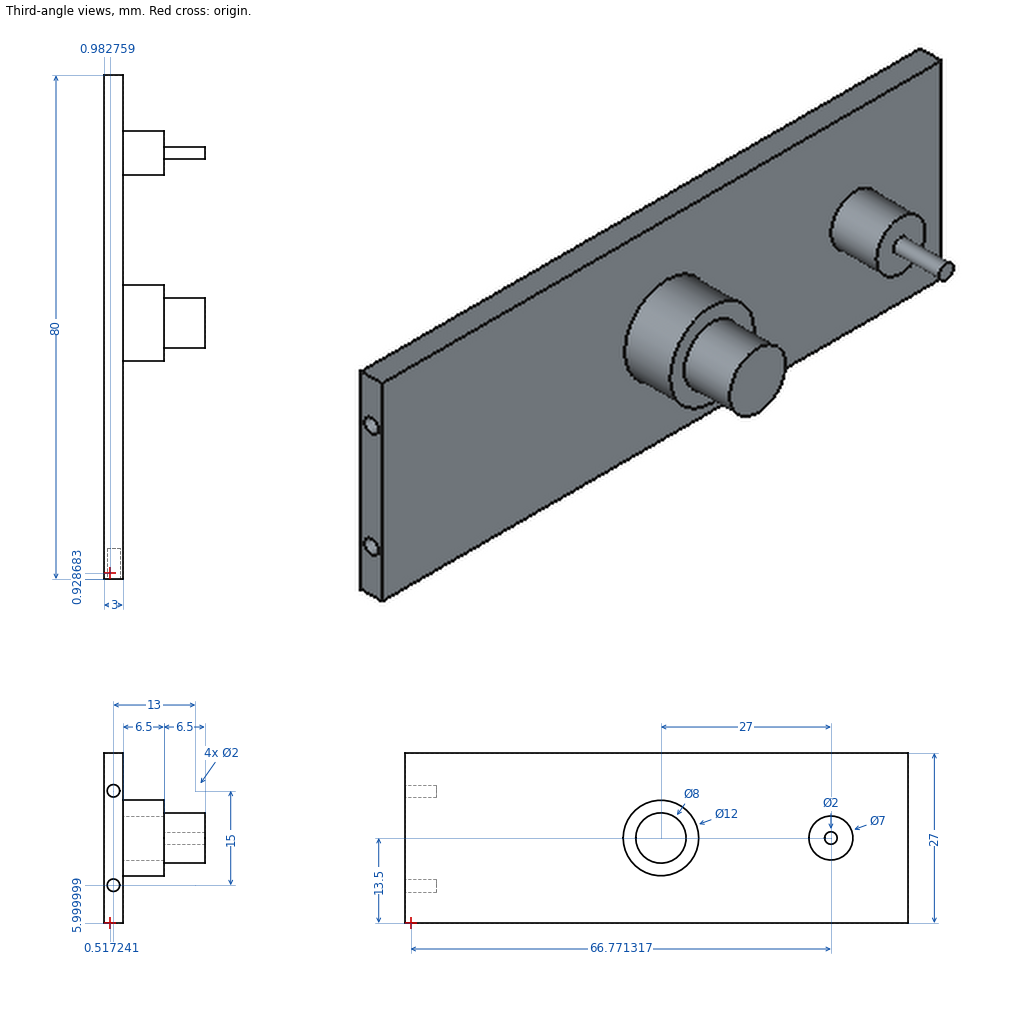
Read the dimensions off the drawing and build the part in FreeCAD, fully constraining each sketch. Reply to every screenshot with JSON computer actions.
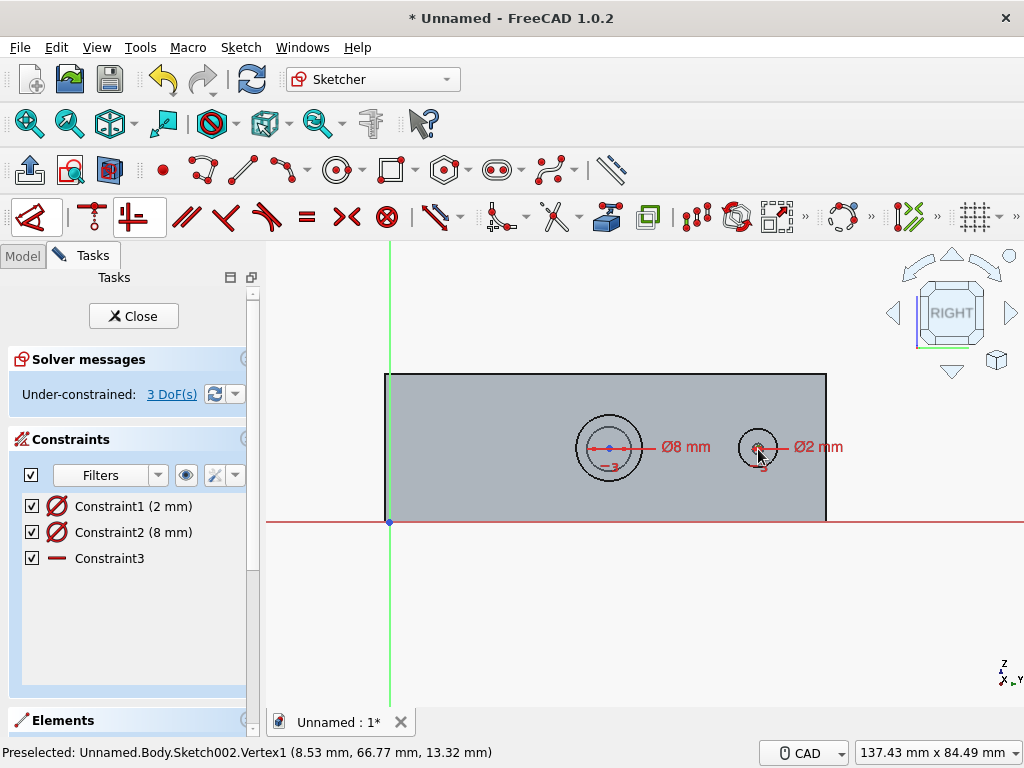
{"action": "left_click", "coordinate": [609, 449]}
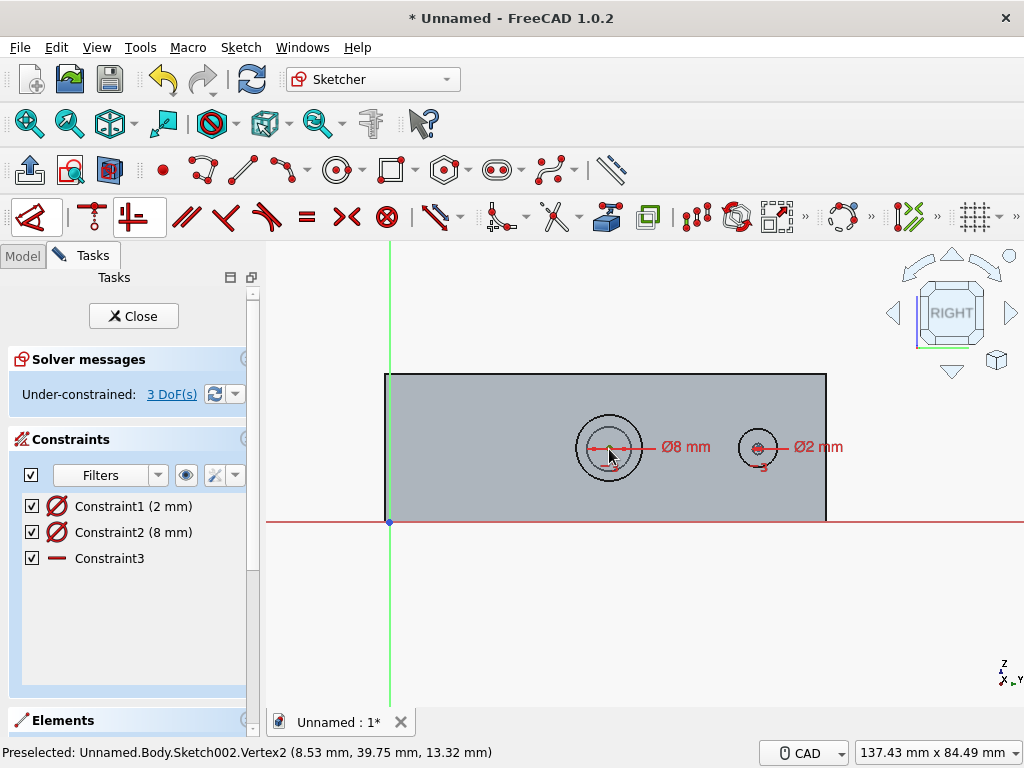
{"action": "left_click", "coordinate": [56, 218]}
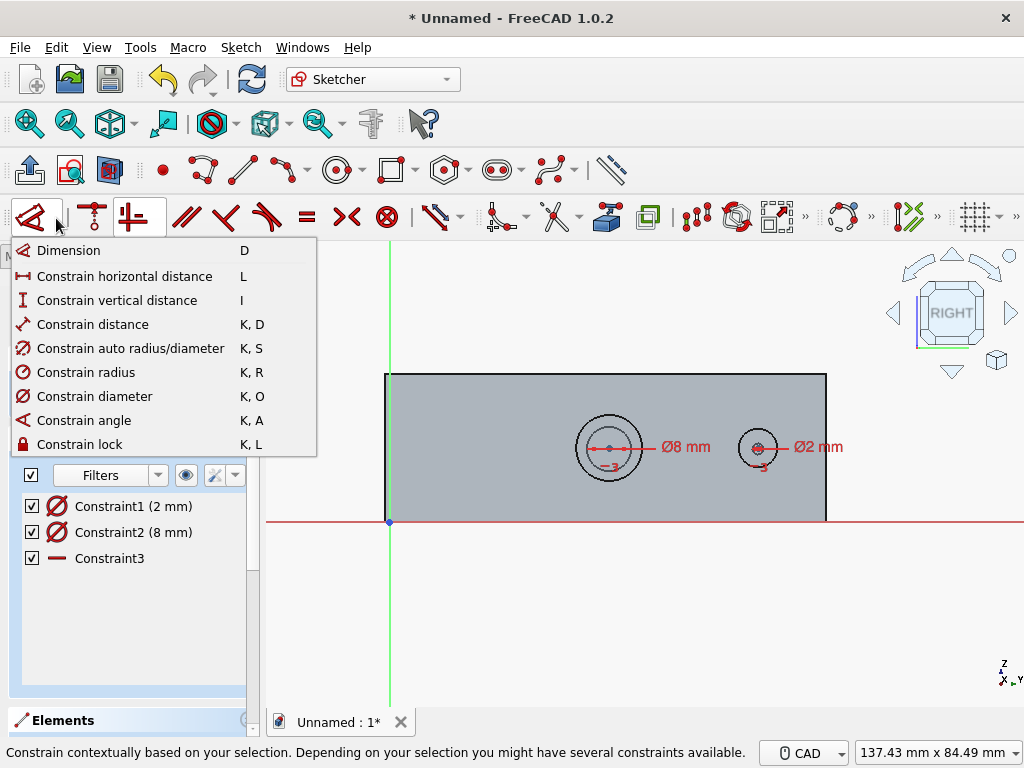
{"action": "left_click", "coordinate": [164, 276]}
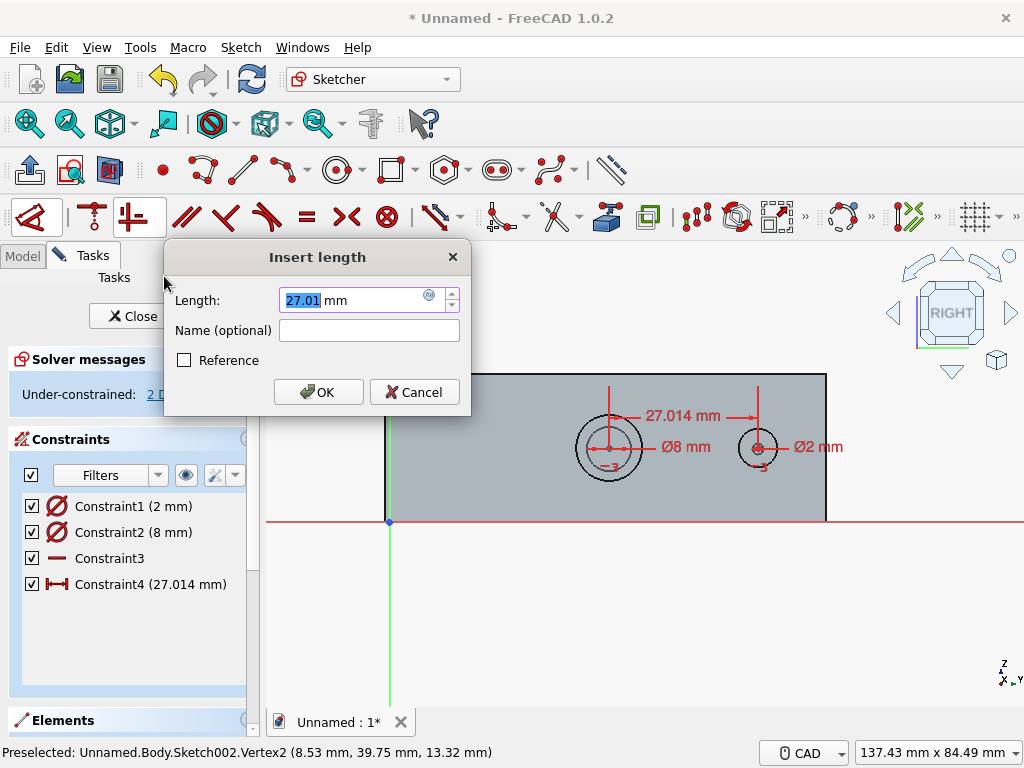
{"action": "type", "text": "27"}
{"action": "key", "text": "Return"}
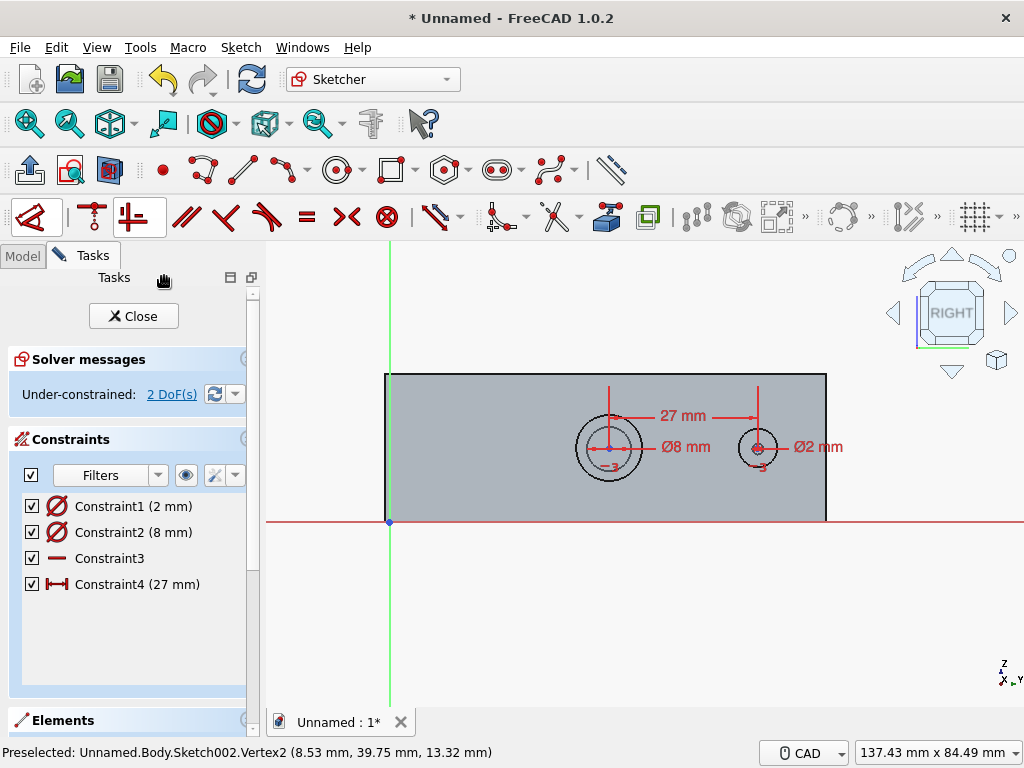
{"action": "left_click", "coordinate": [758, 449]}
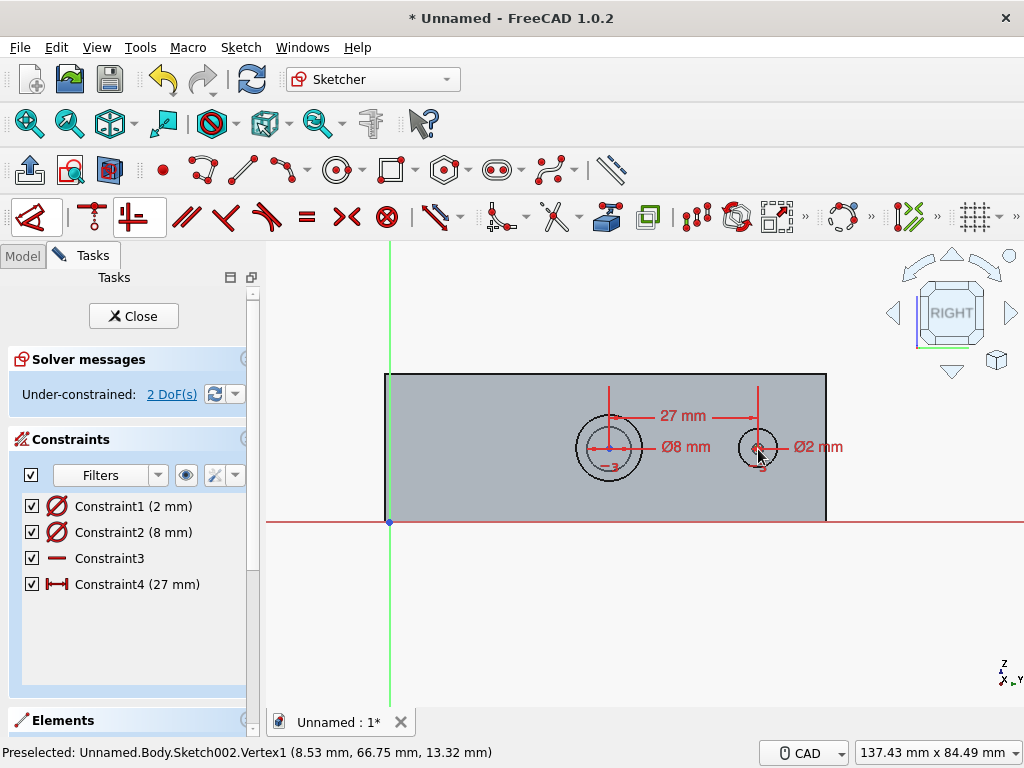
{"action": "key", "text": "i"}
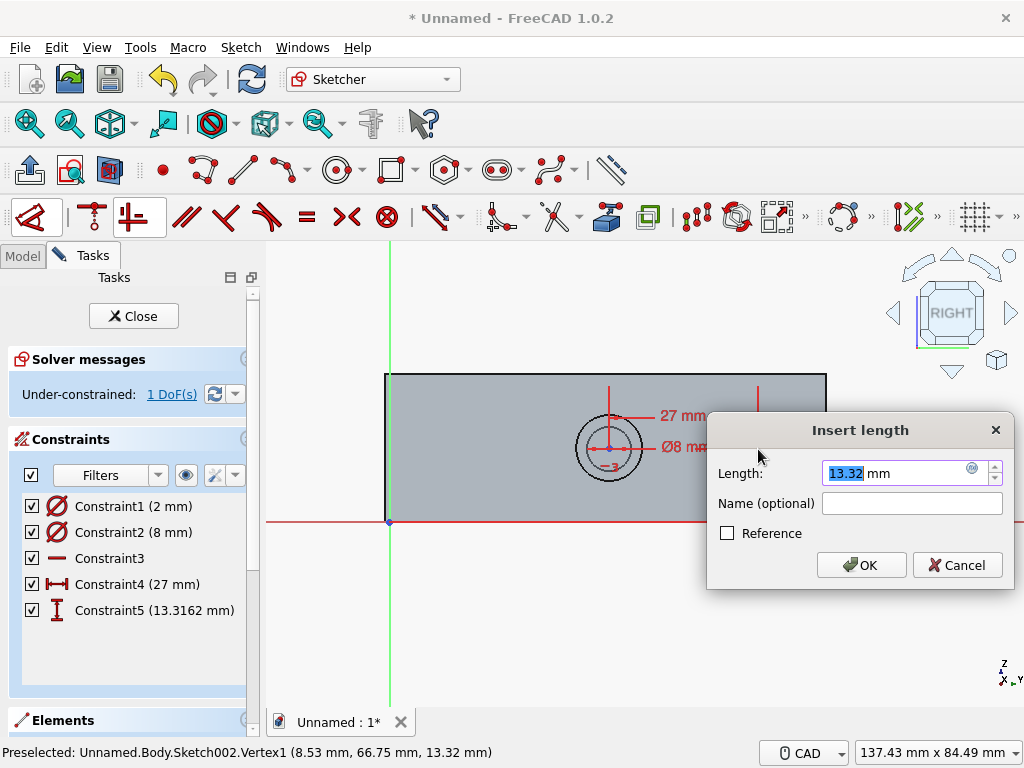
{"action": "type", "text": "13.5"}
{"action": "key", "text": "Return"}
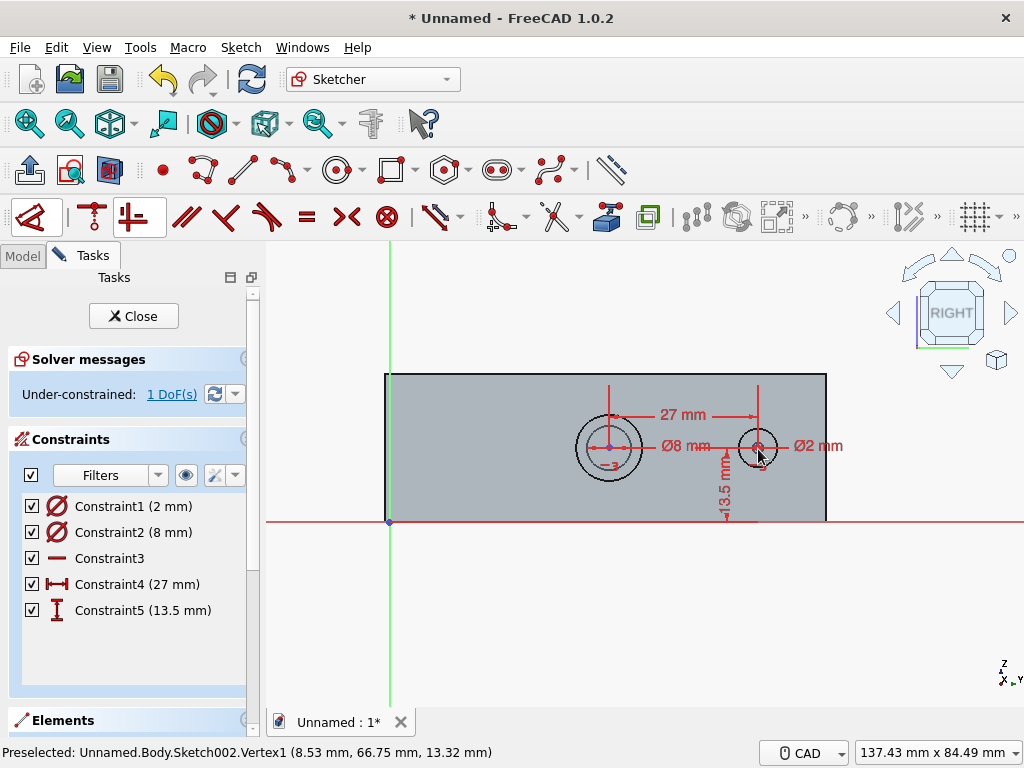
{"action": "left_click", "coordinate": [758, 448]}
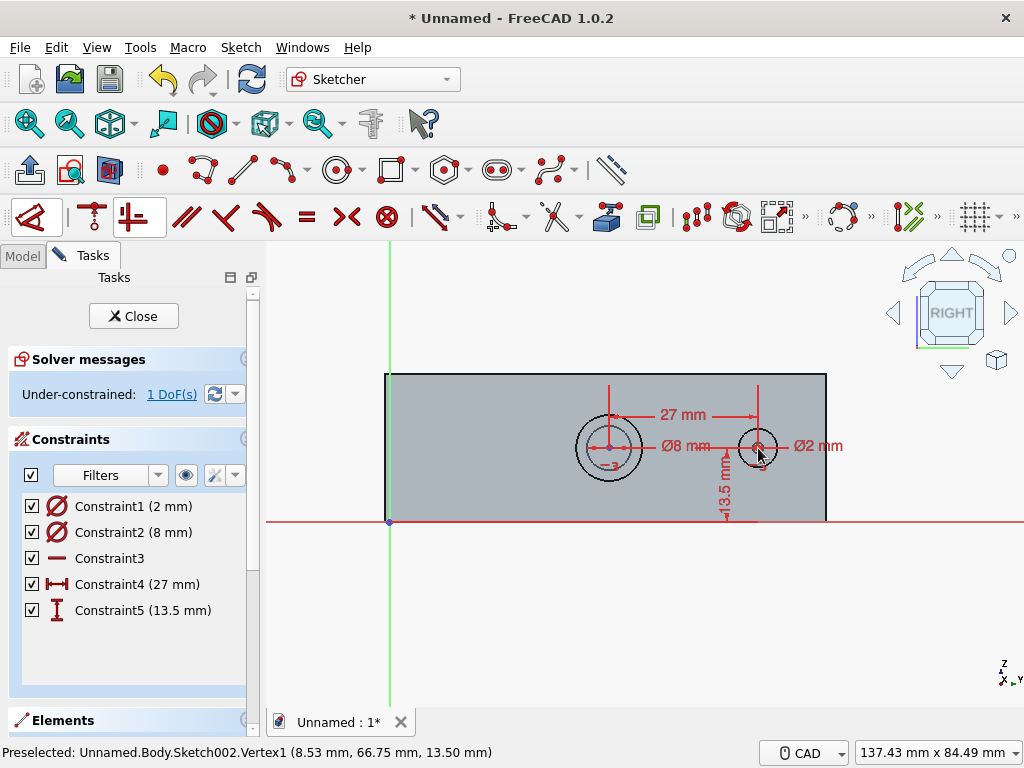
{"action": "left_click", "coordinate": [56, 218]}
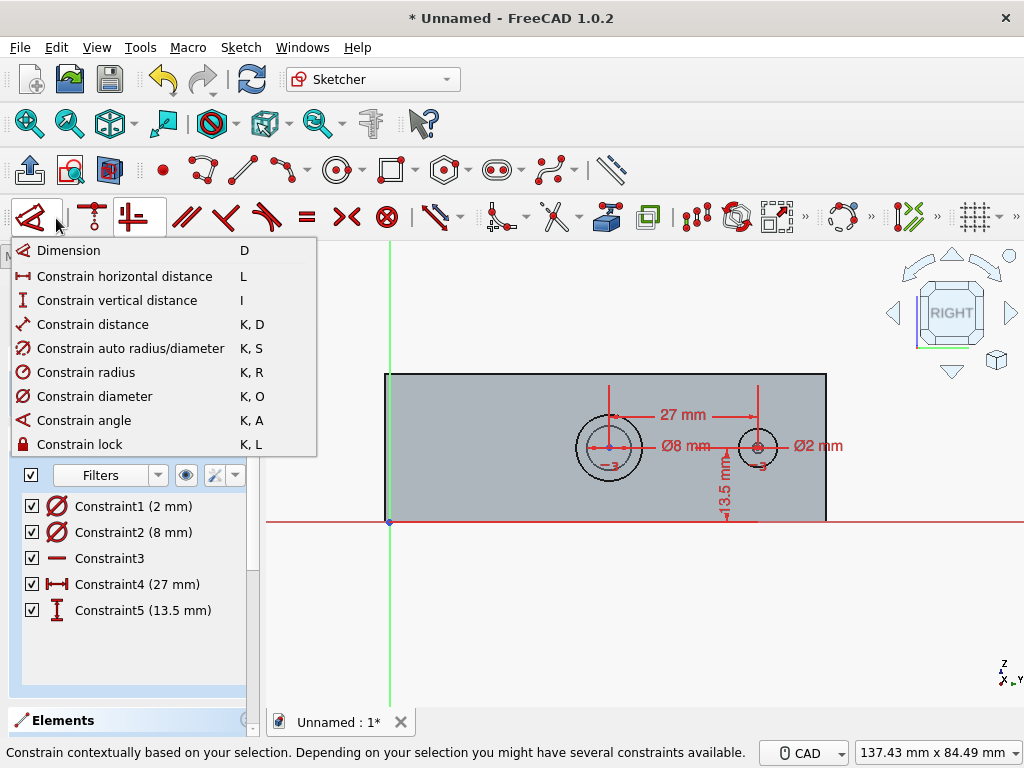
{"action": "left_click", "coordinate": [164, 276]}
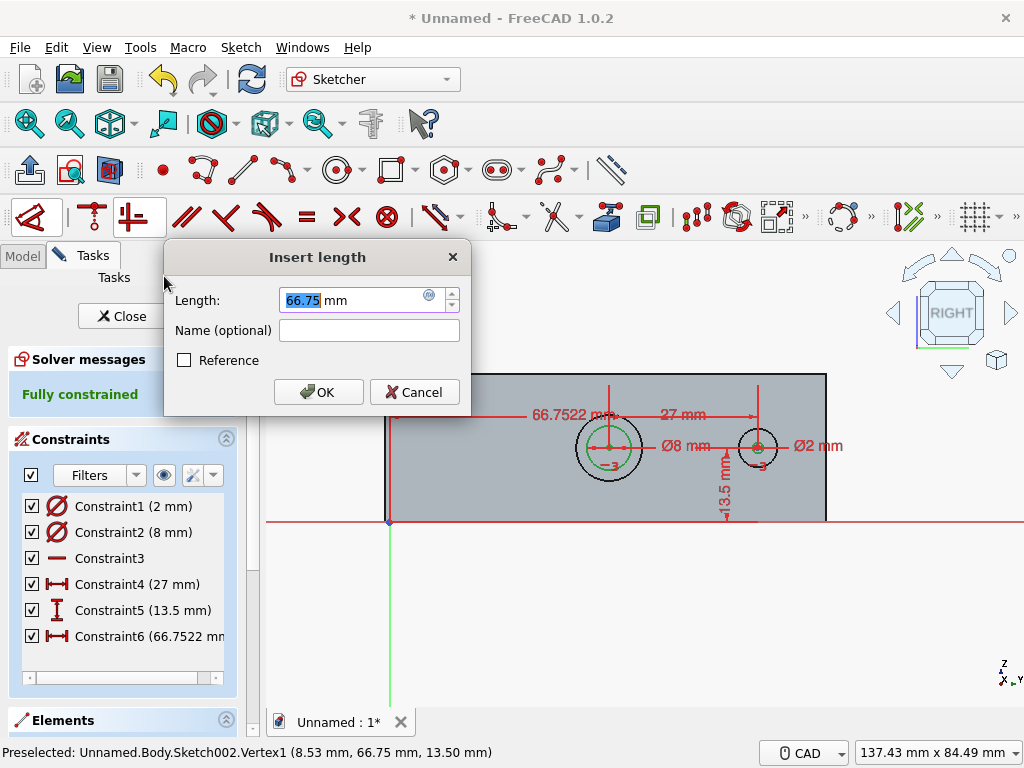
{"action": "type", "text": "66.771317"}
{"action": "key", "text": "Return"}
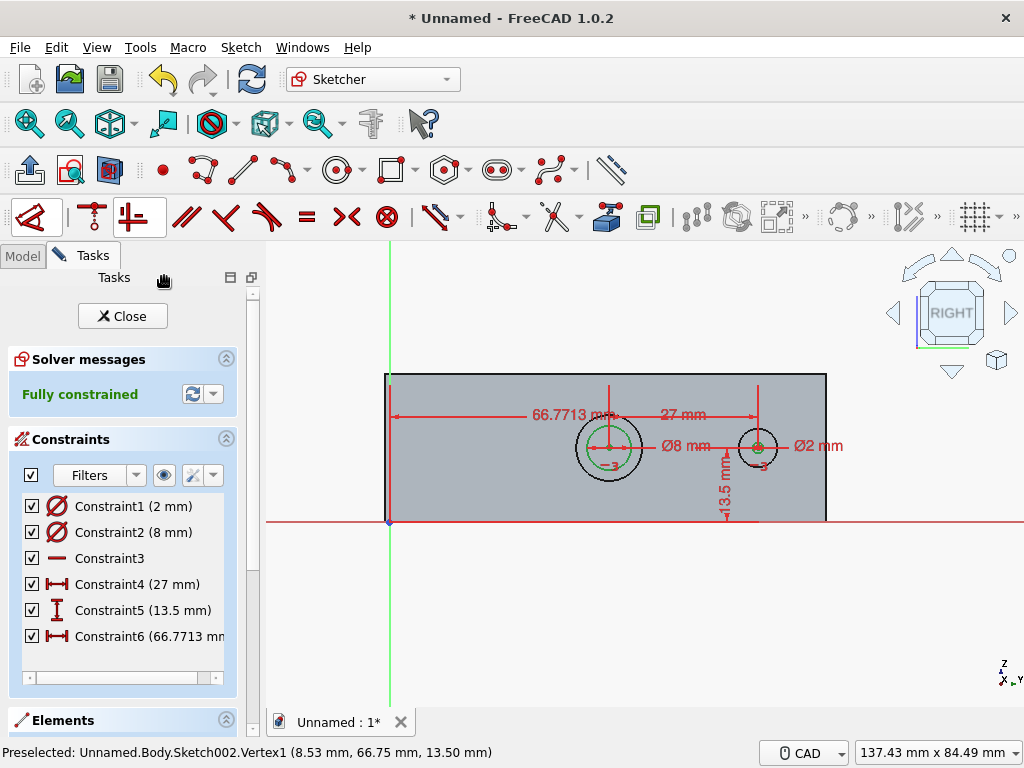
{"action": "left_click", "coordinate": [123, 316]}